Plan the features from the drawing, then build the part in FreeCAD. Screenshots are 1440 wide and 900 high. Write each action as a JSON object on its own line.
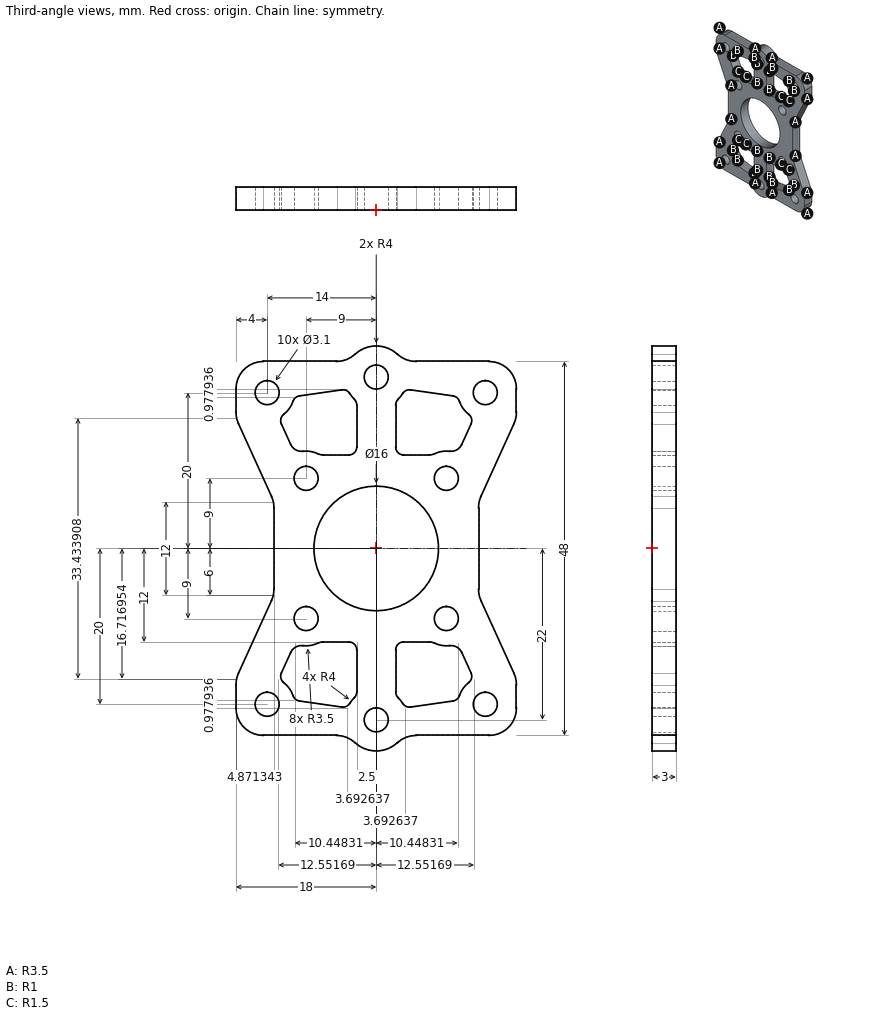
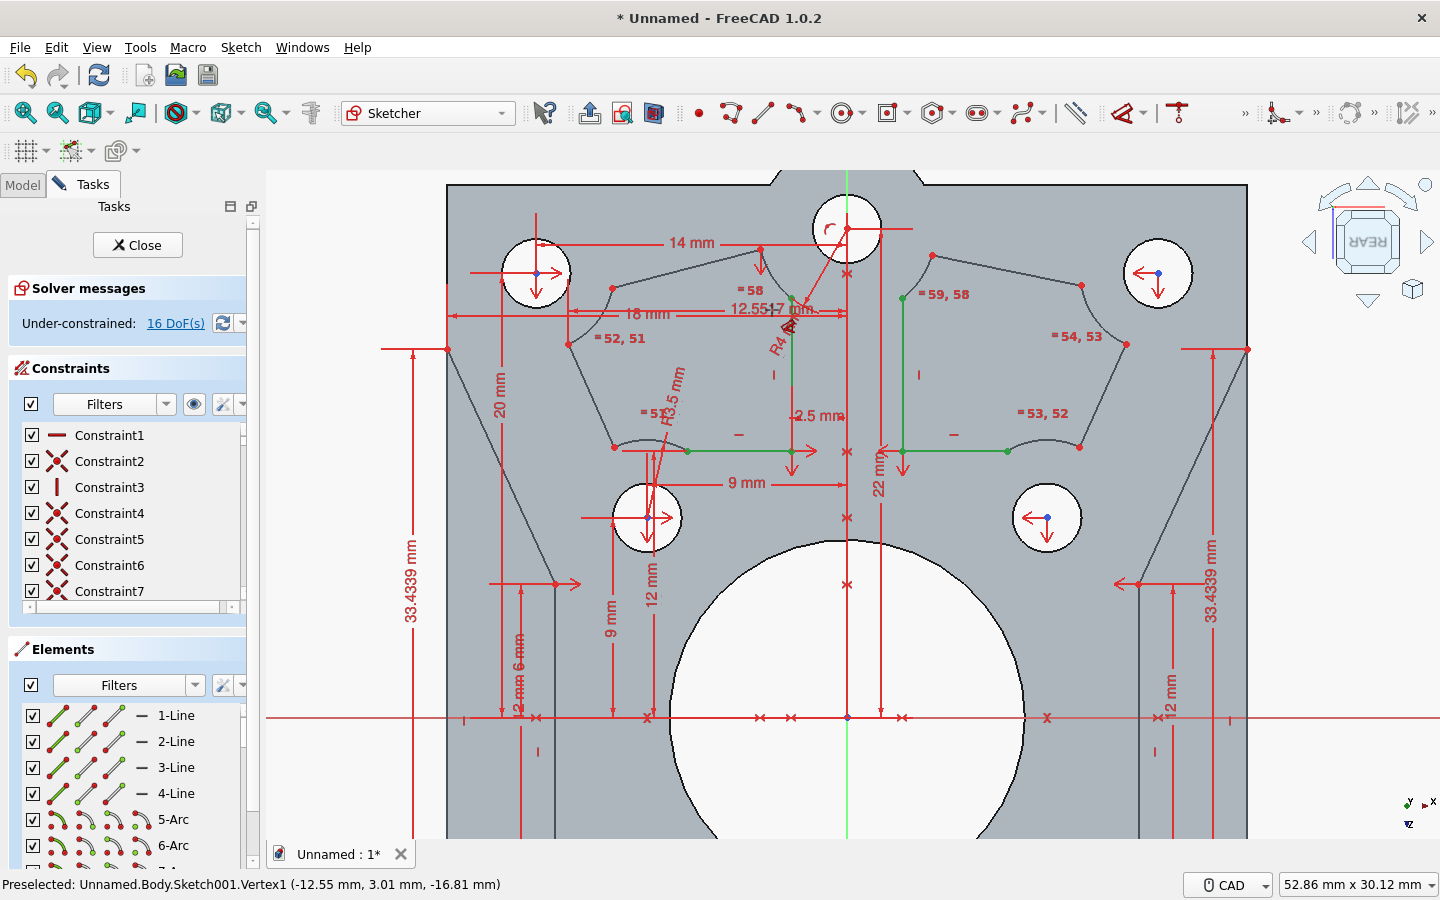
{"action": "left_click", "coordinate": [614, 447]}
{"action": "left_click", "coordinate": [731, 752]}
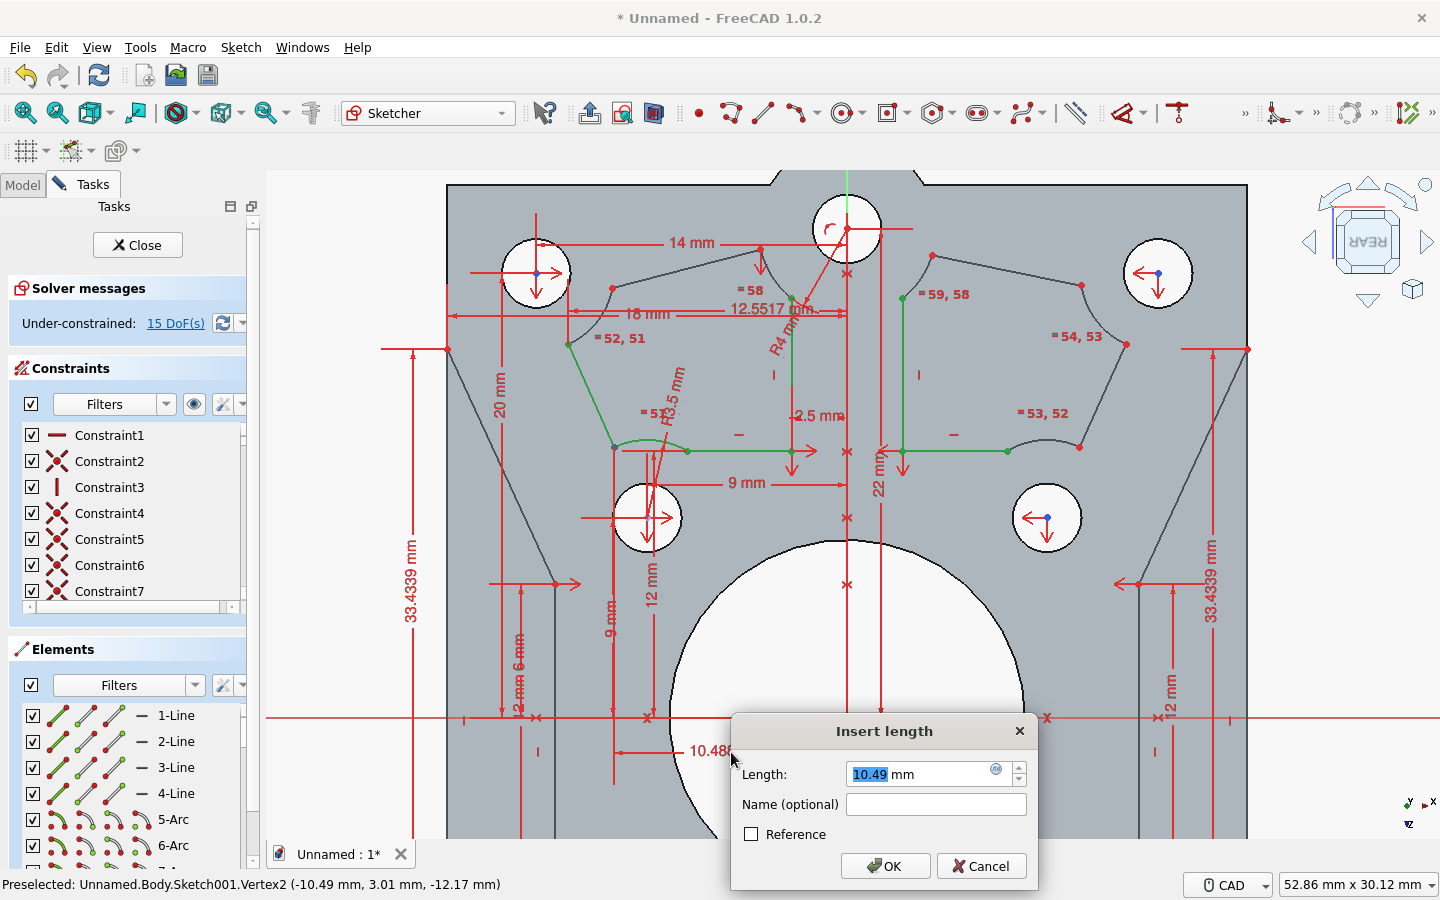
{"action": "type", "text": "10.44831"}
{"action": "key", "text": "Return"}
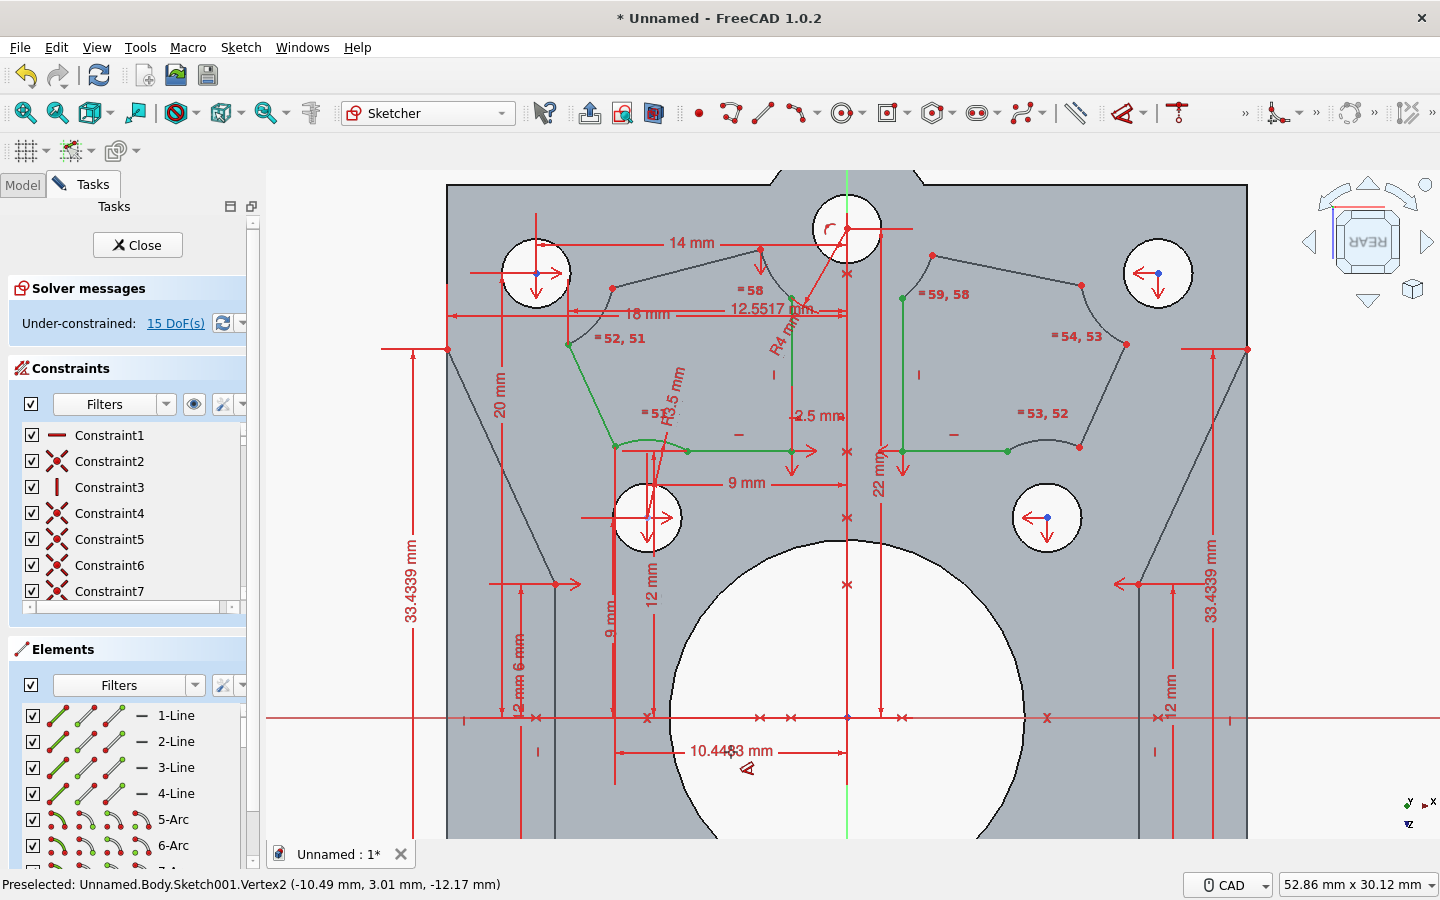
{"action": "left_click", "coordinate": [761, 250]}
{"action": "left_click", "coordinate": [804, 216]}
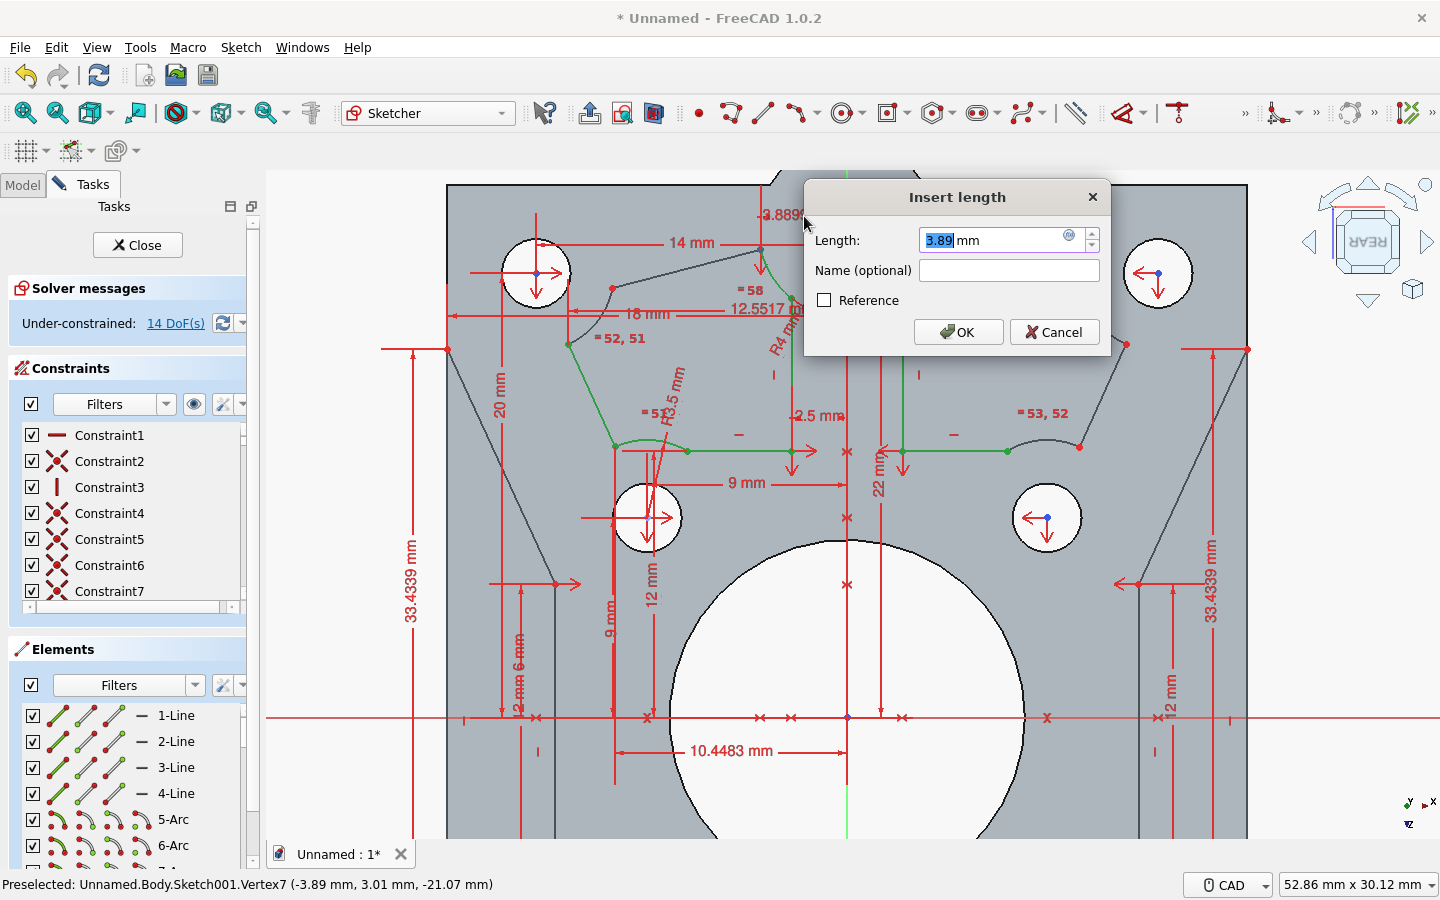
{"action": "type", "text": "3.692637"}
{"action": "key", "text": "Return"}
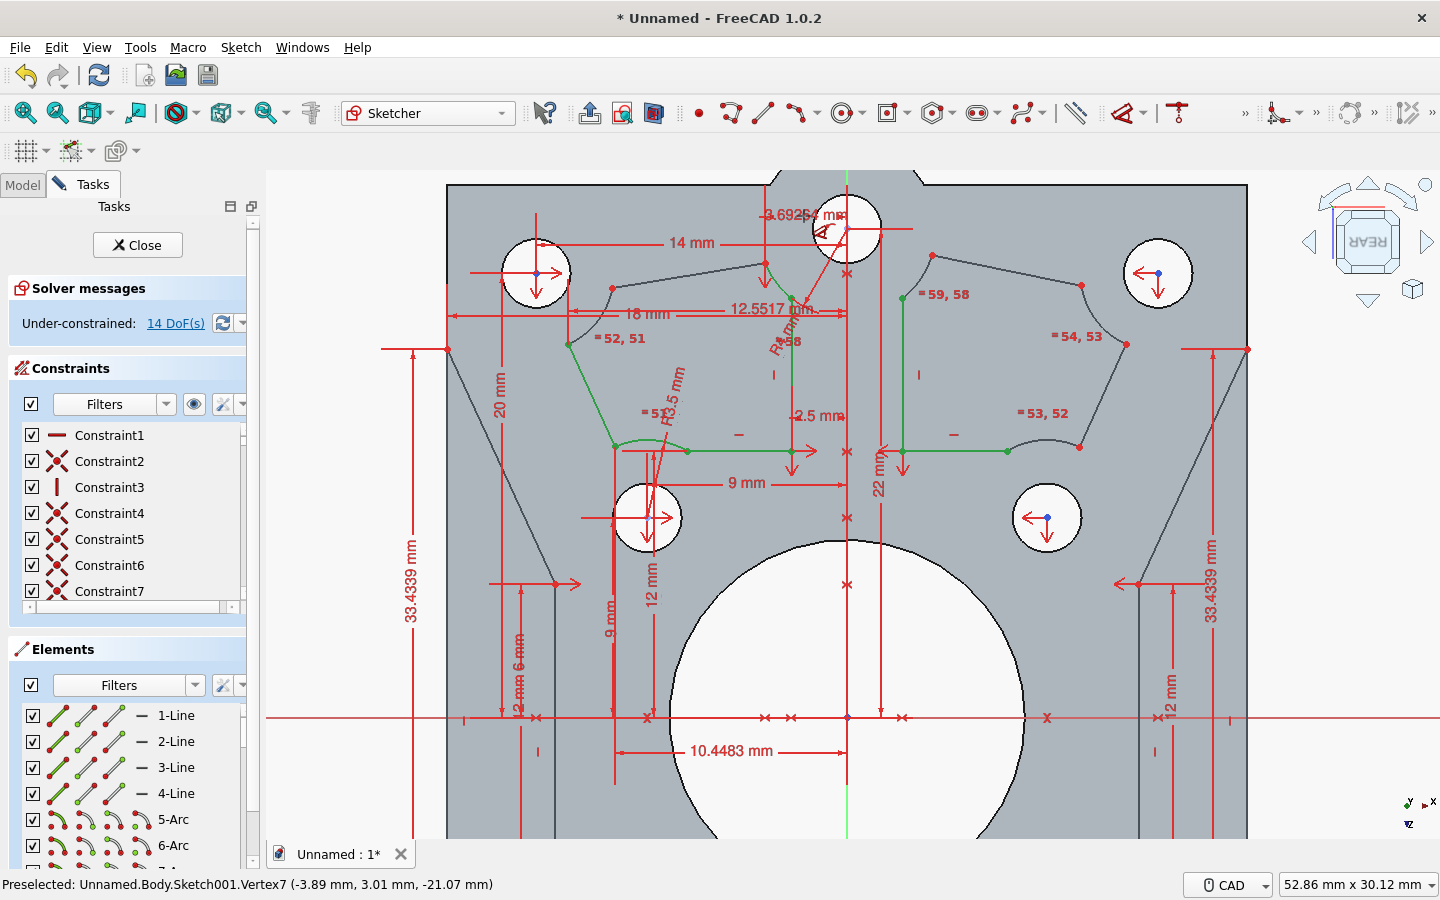
{"action": "left_click", "coordinate": [1080, 447]}
{"action": "left_click", "coordinate": [963, 413]}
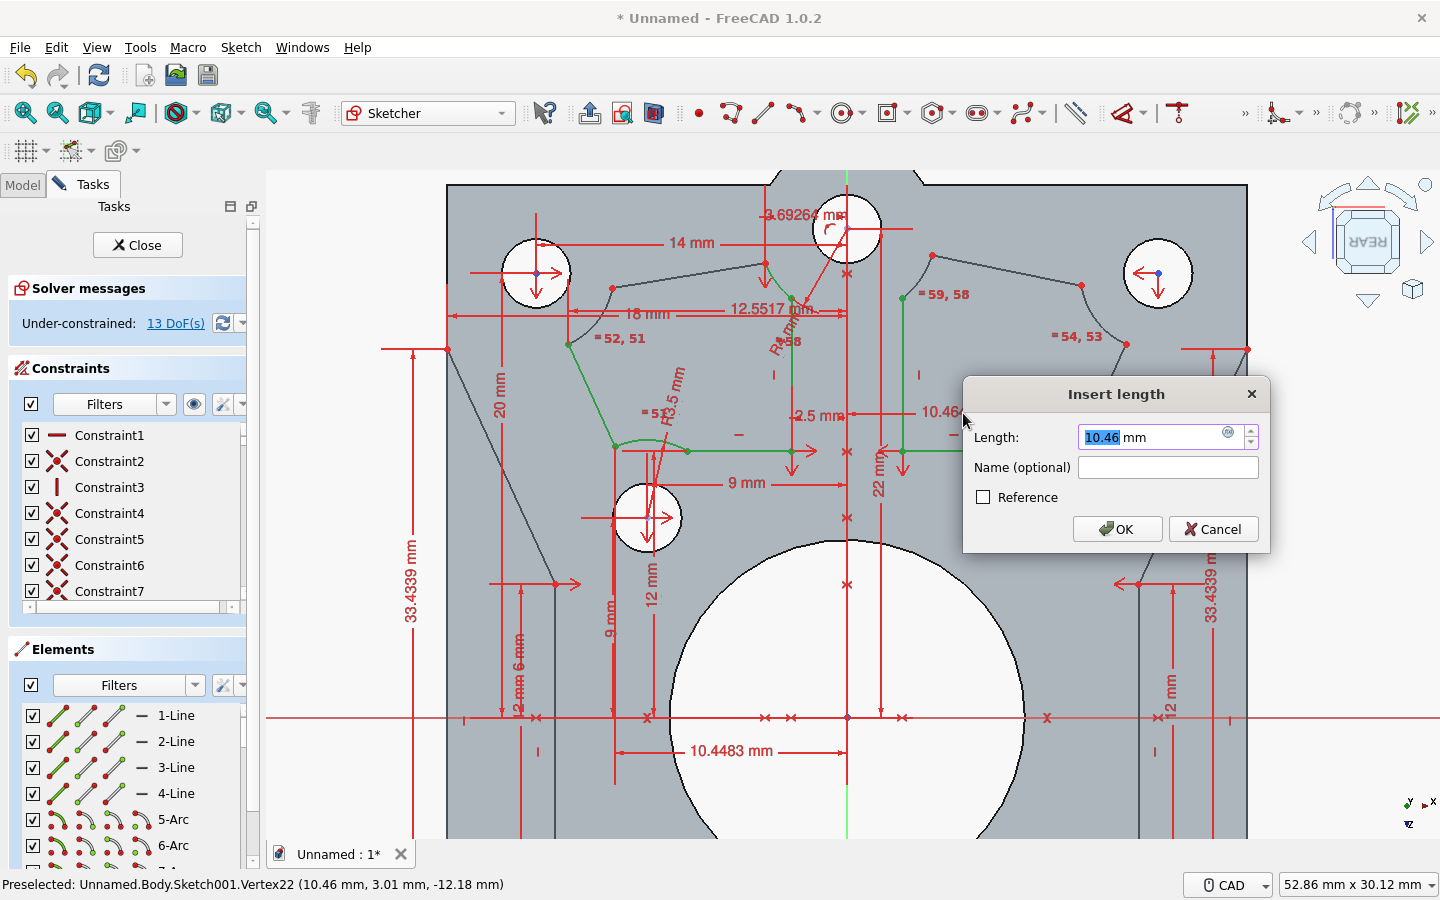
{"action": "type", "text": "10.44831"}
{"action": "key", "text": "Return"}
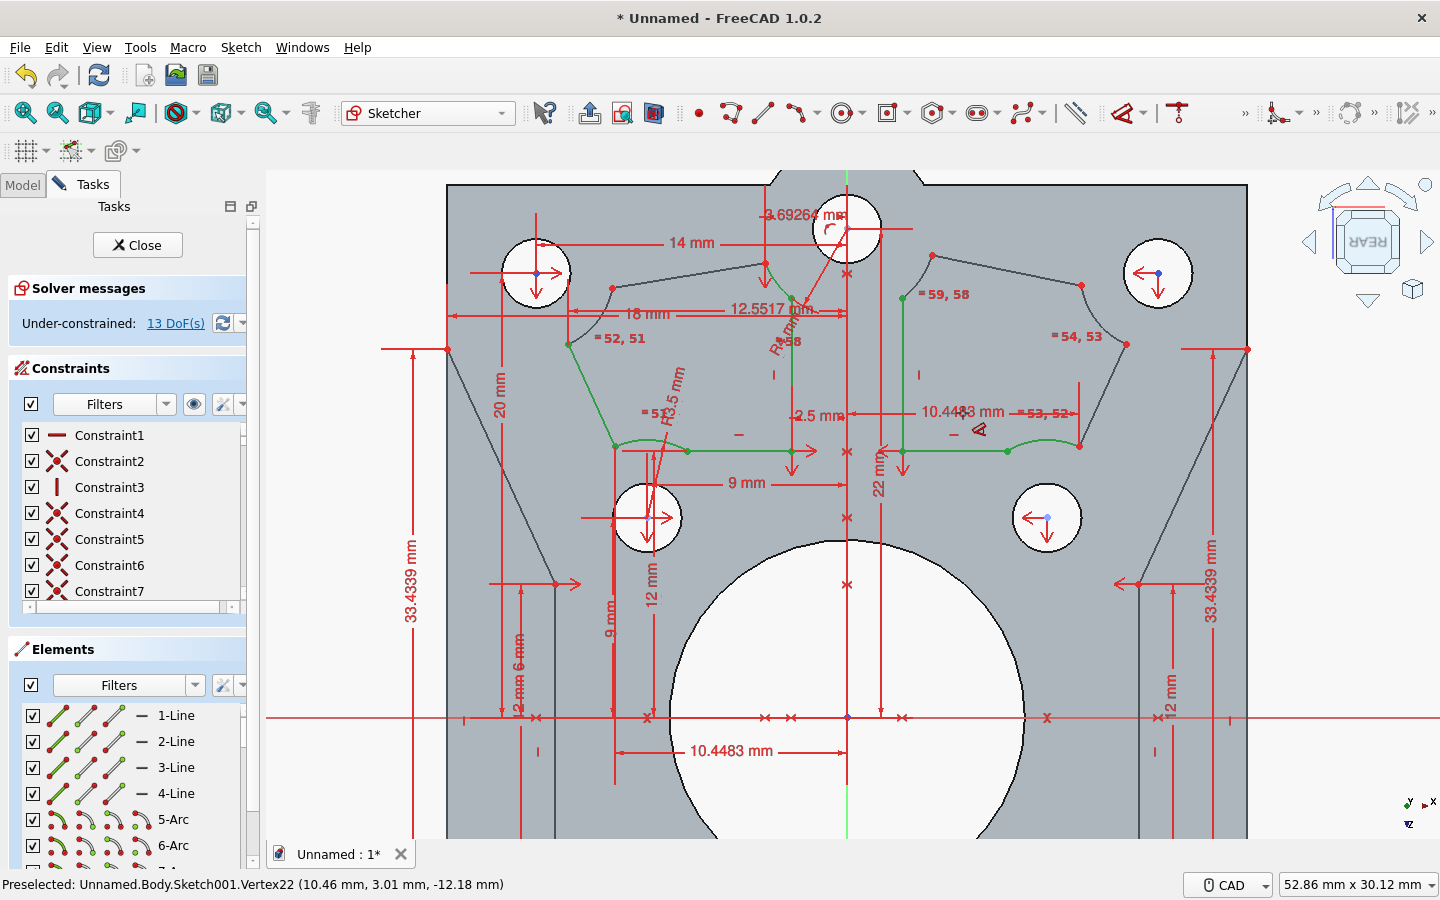
{"action": "left_click", "coordinate": [1126, 344]}
{"action": "left_click", "coordinate": [987, 310]}